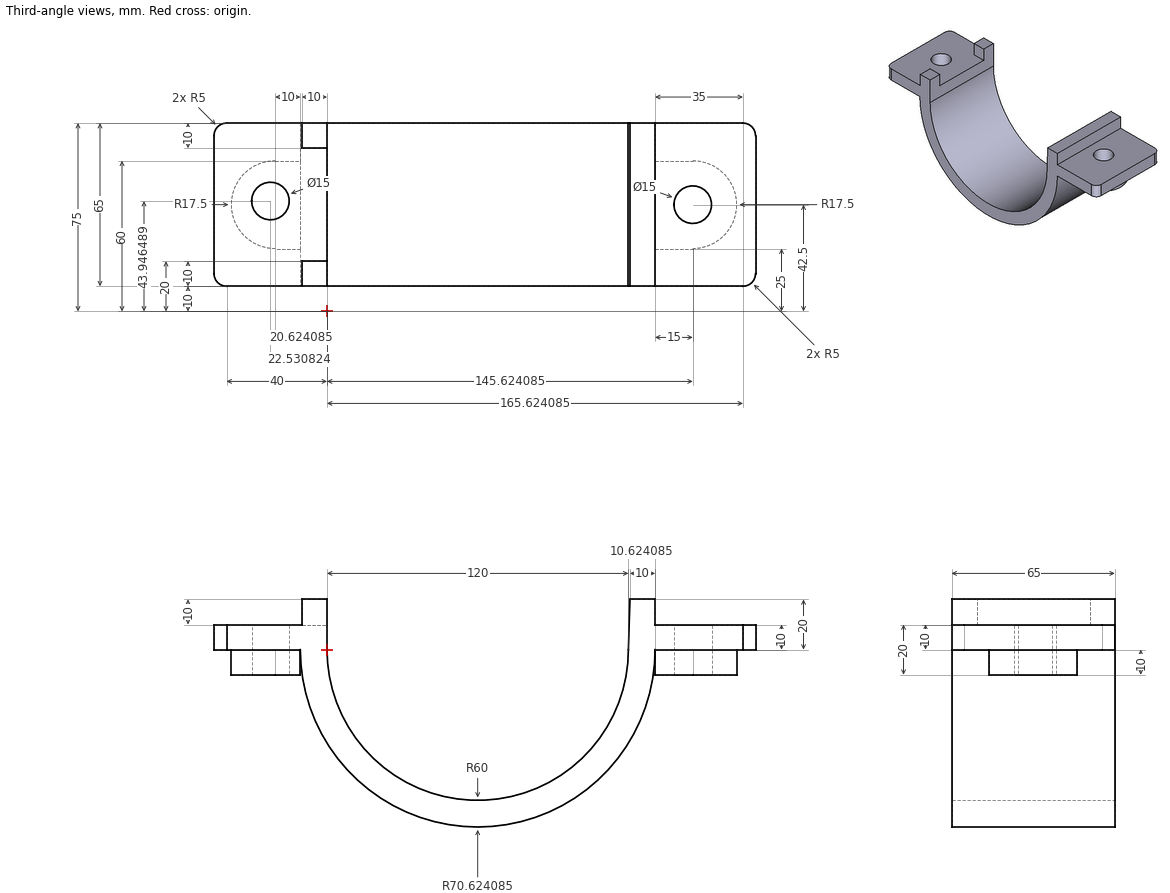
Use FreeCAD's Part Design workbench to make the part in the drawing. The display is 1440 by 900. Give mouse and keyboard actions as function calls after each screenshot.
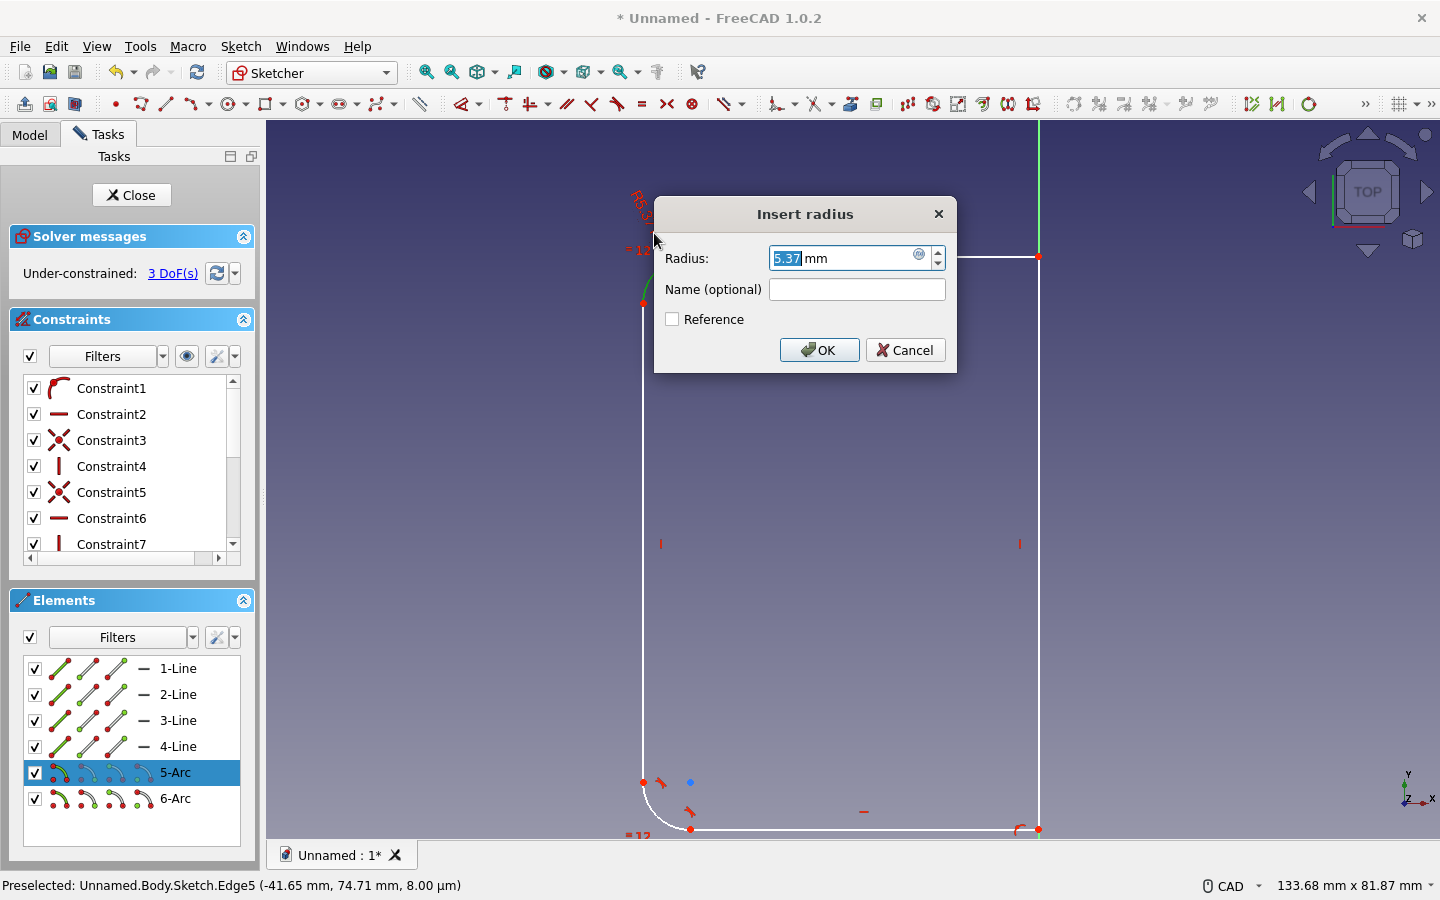
text(5)
key(Return)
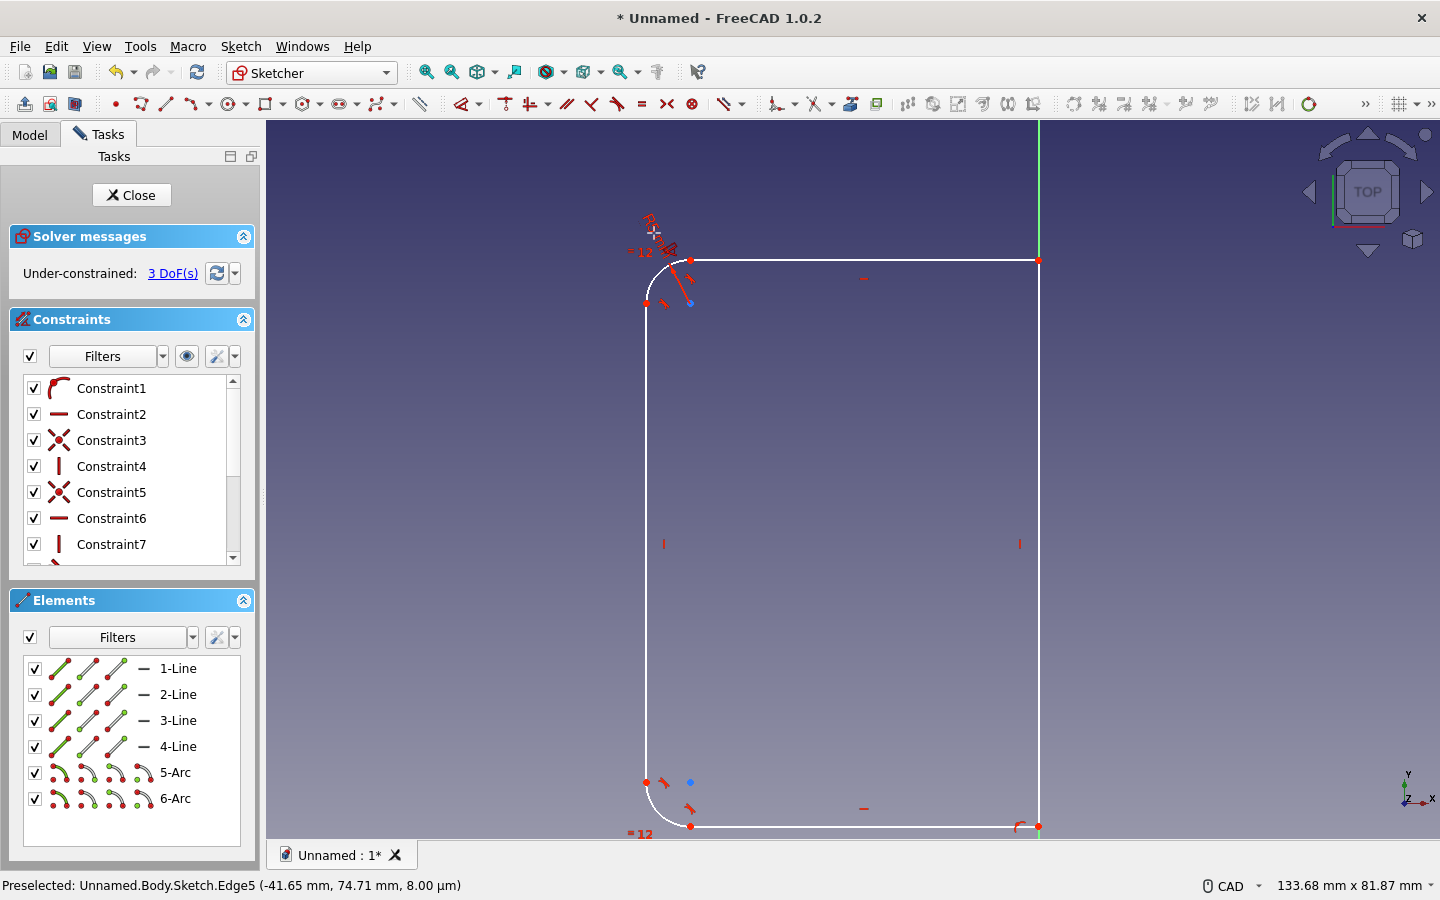
scroll(669, 261, down, 2)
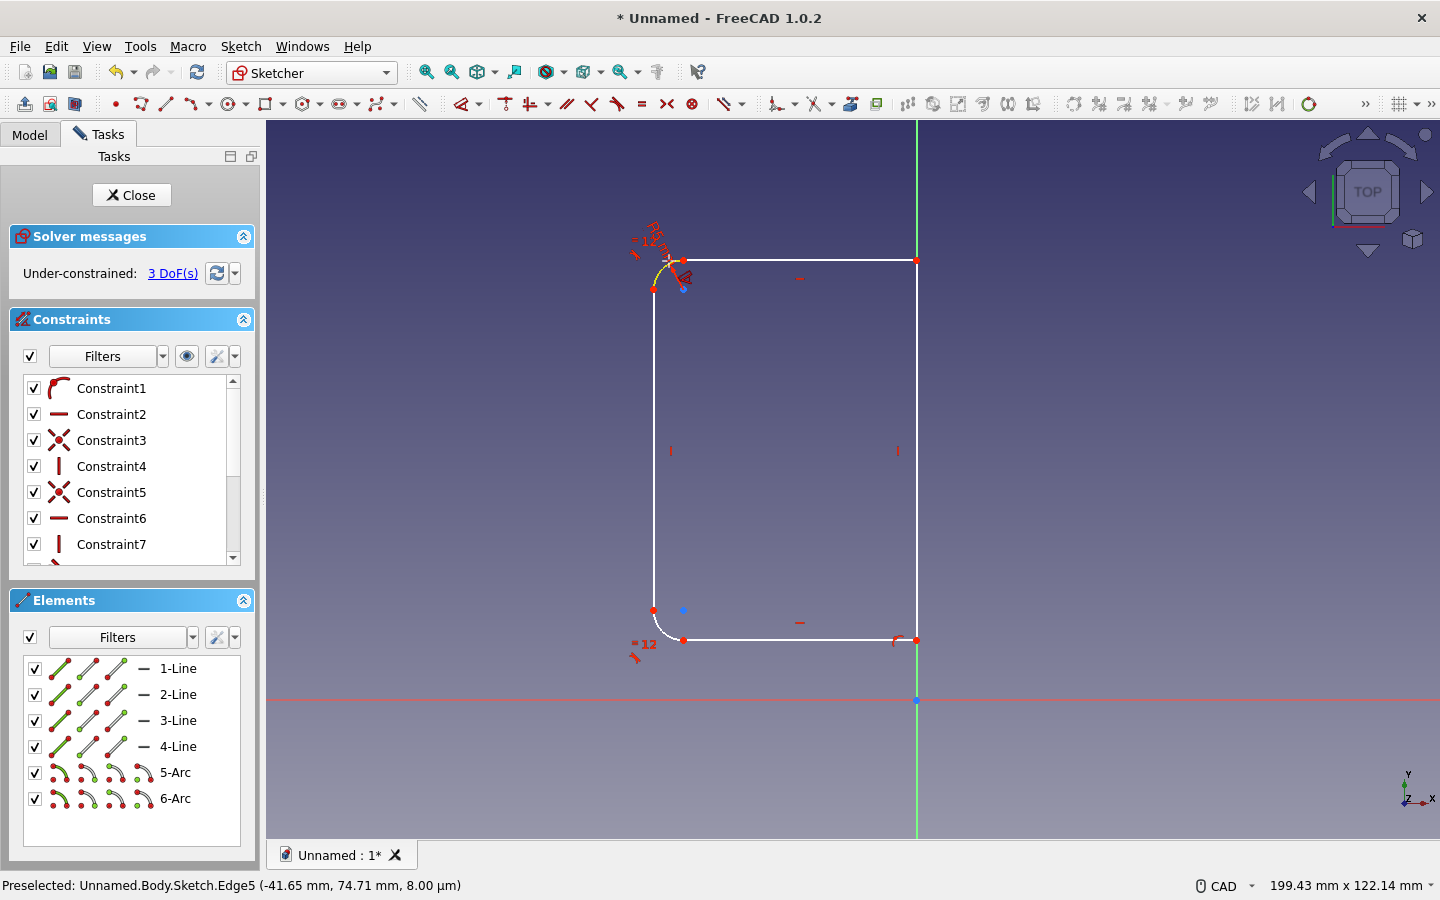
click(753, 640)
click(800, 674)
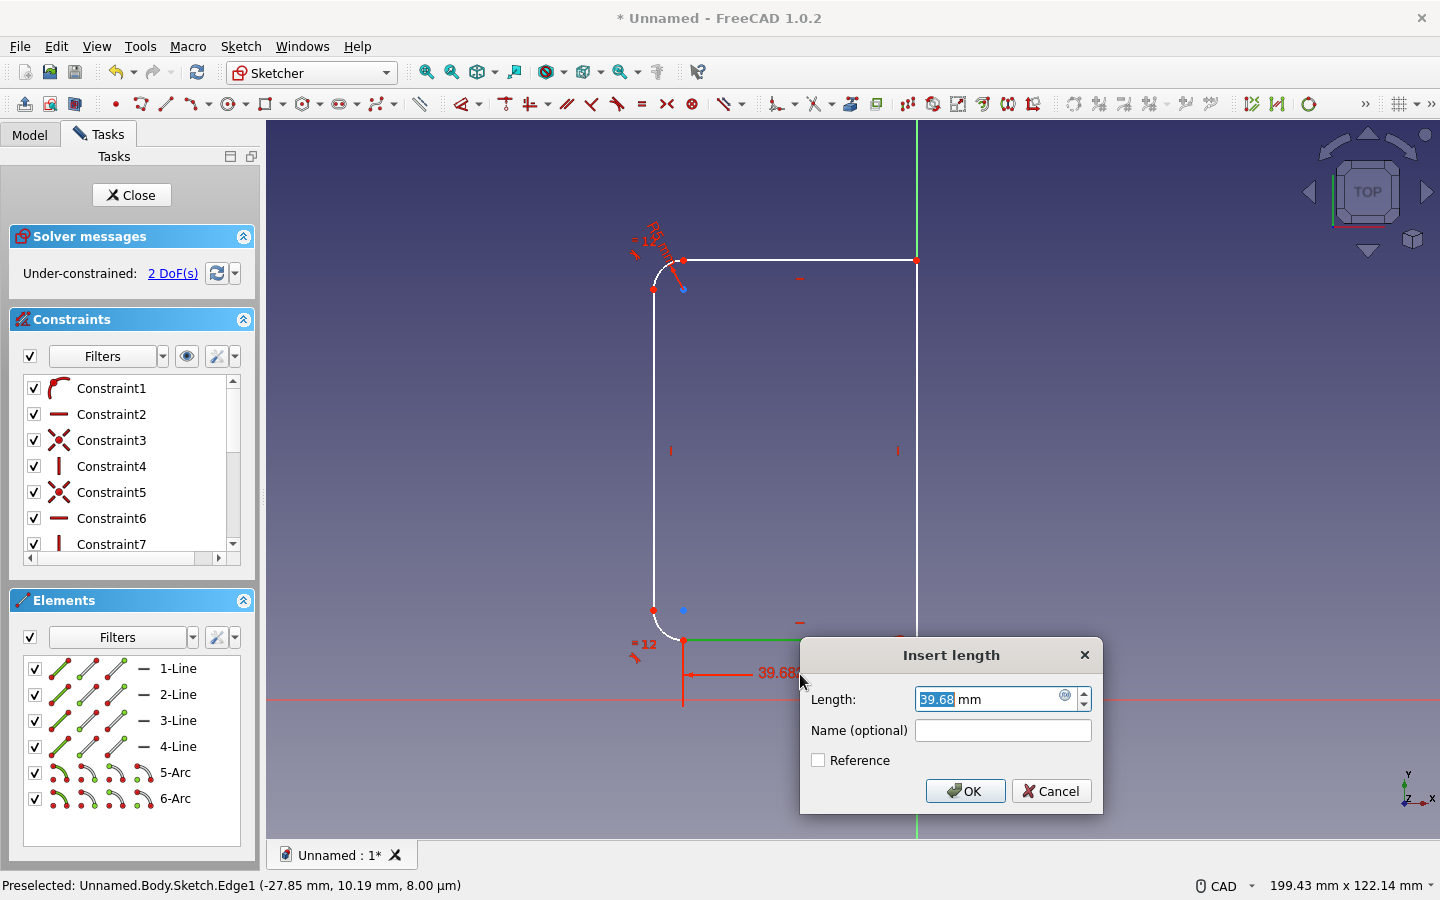
text(40)
key(Return)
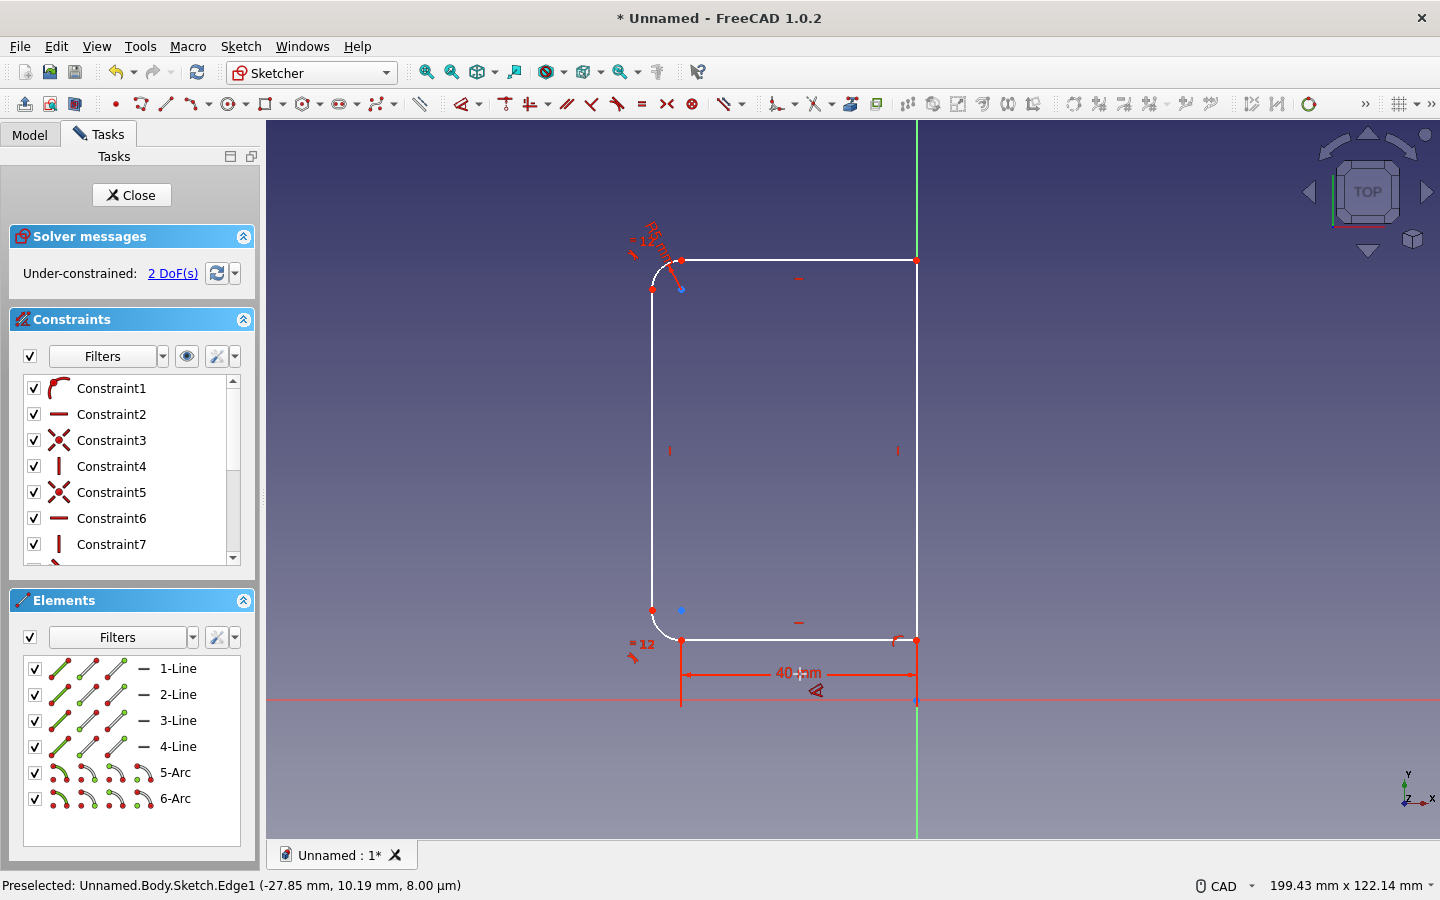
click(917, 526)
click(951, 450)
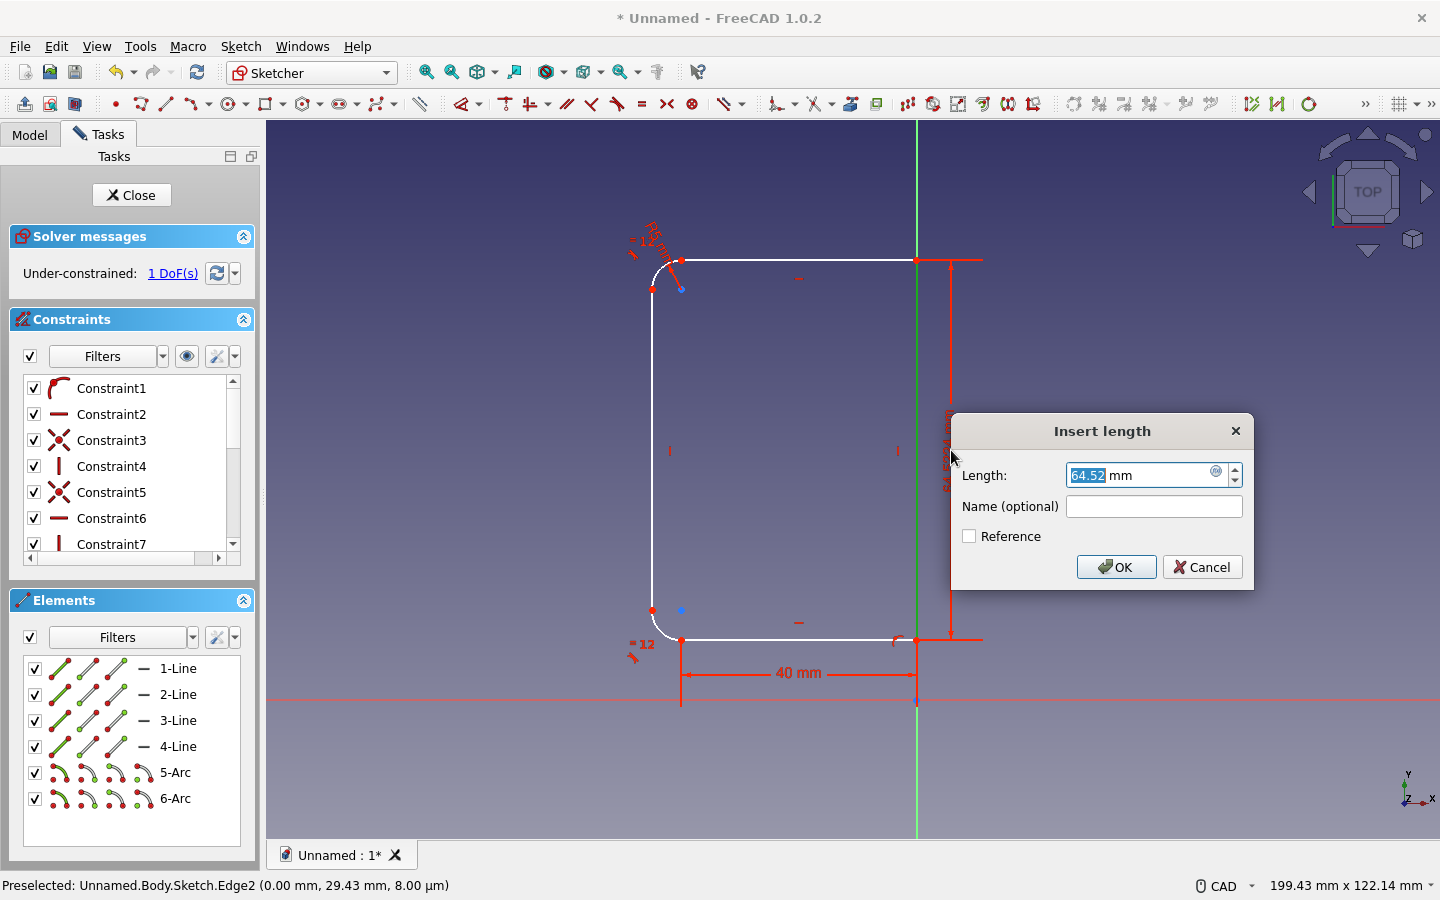
text(65)
key(Return)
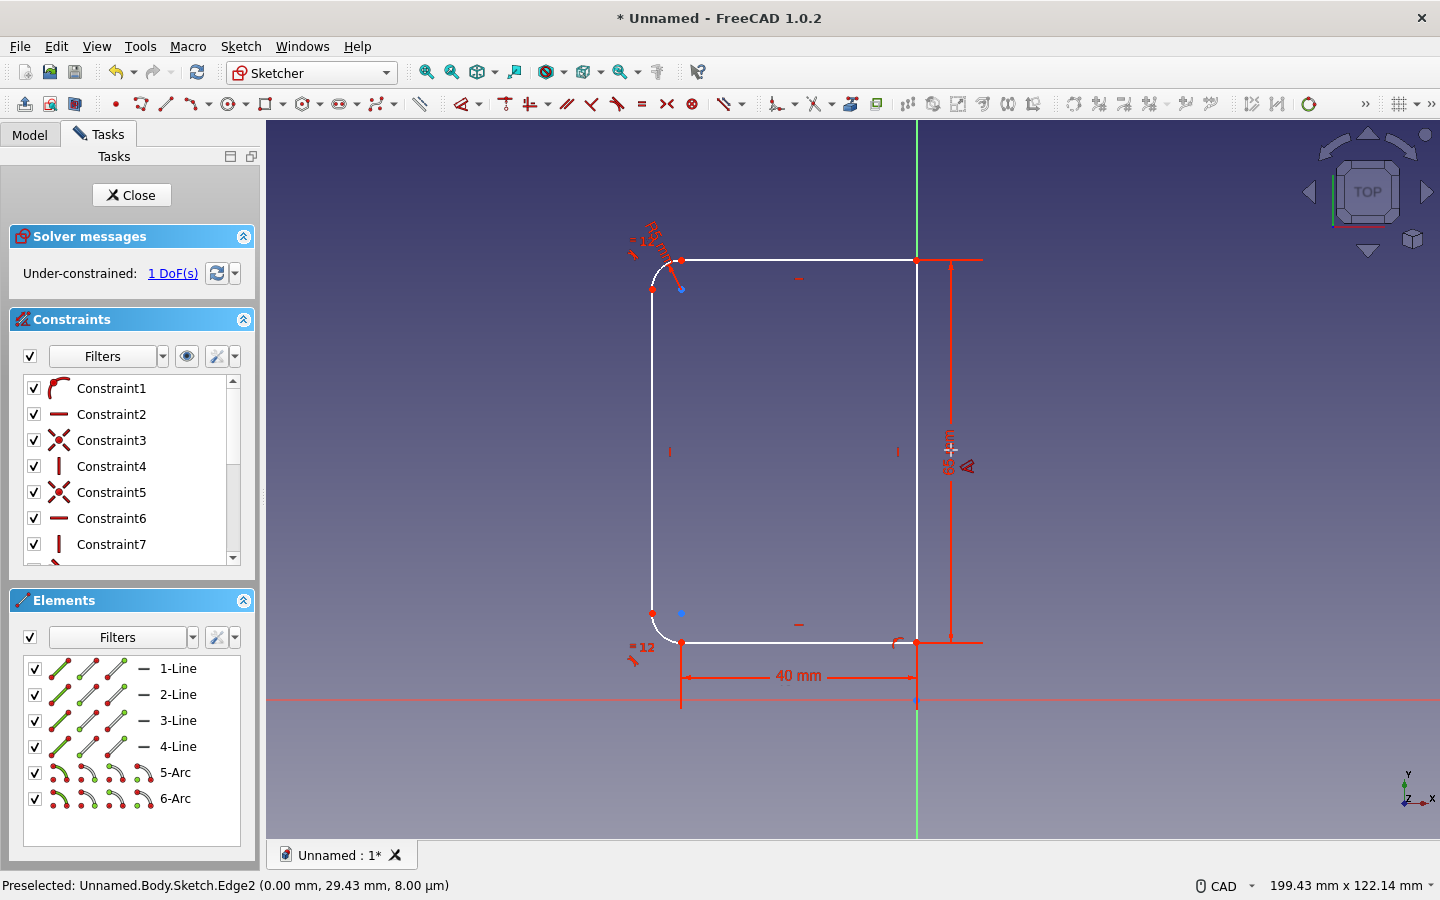
click(681, 643)
click(951, 672)